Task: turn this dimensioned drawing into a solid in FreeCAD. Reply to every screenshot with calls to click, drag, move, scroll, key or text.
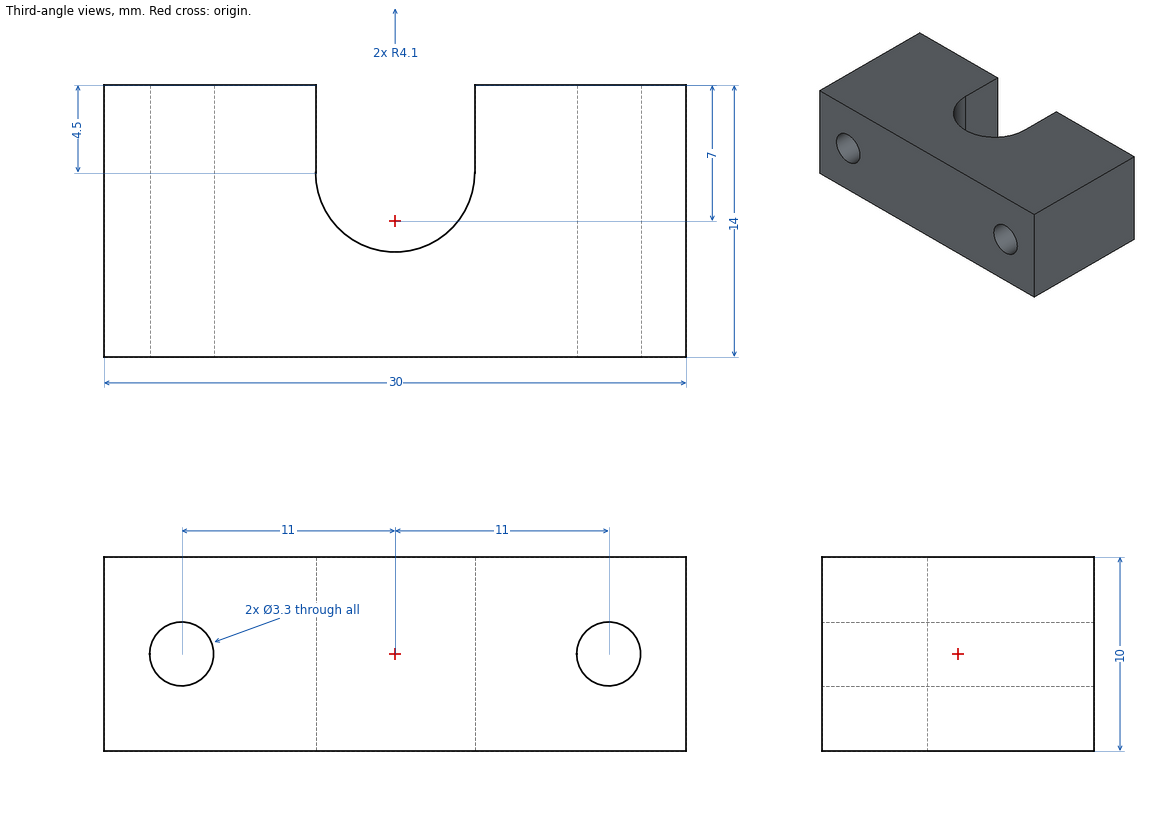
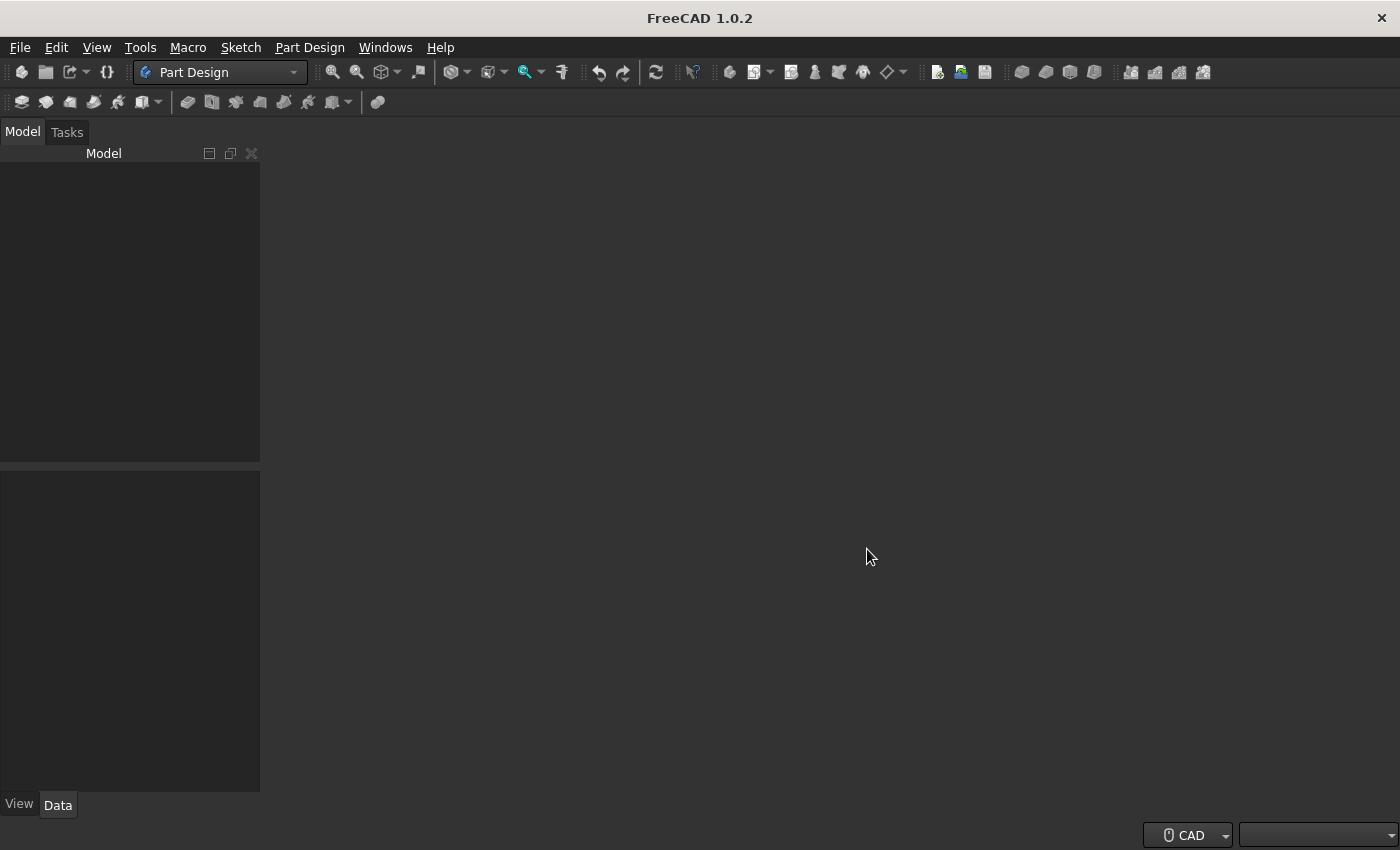
click(938, 72)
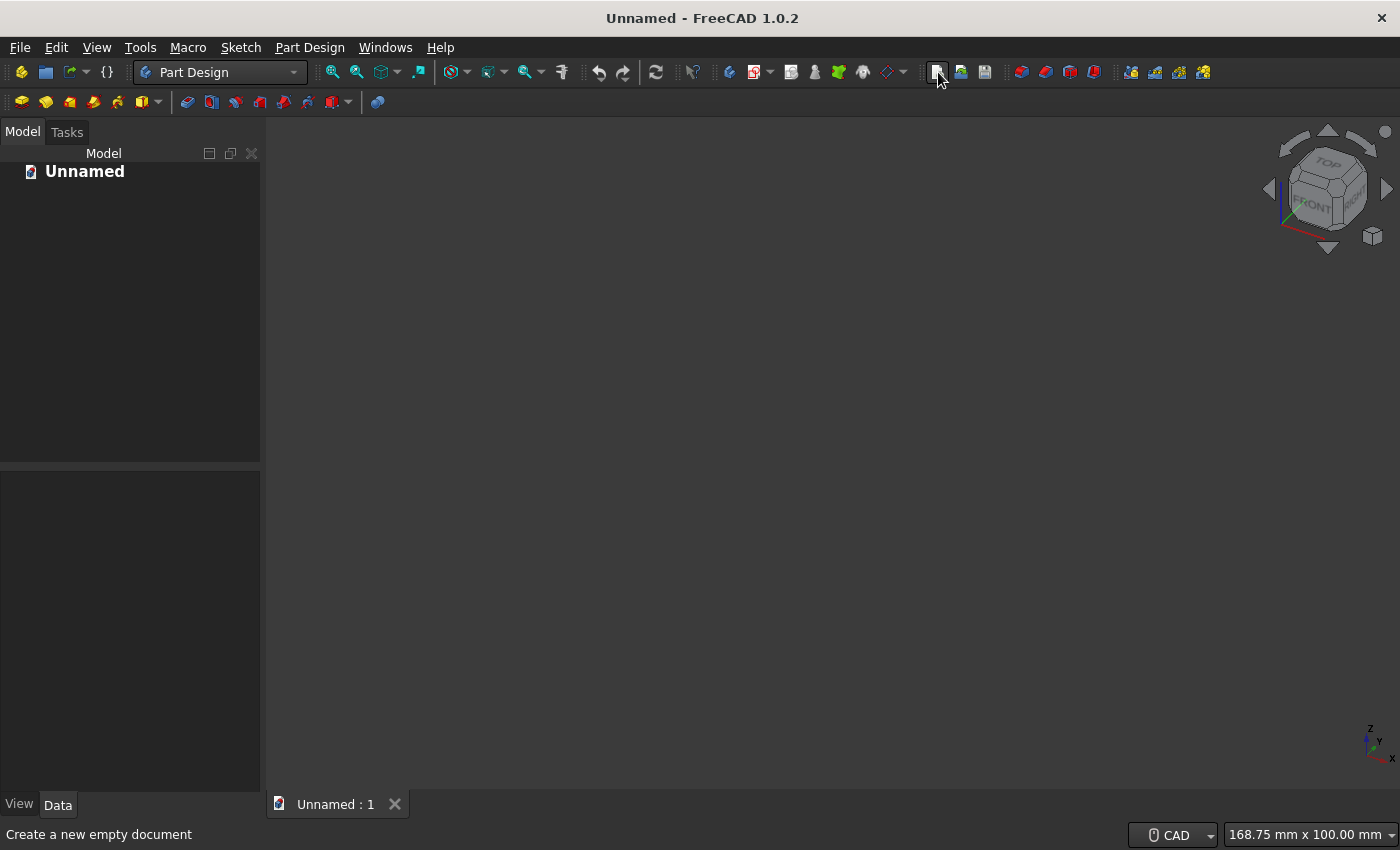
click(754, 72)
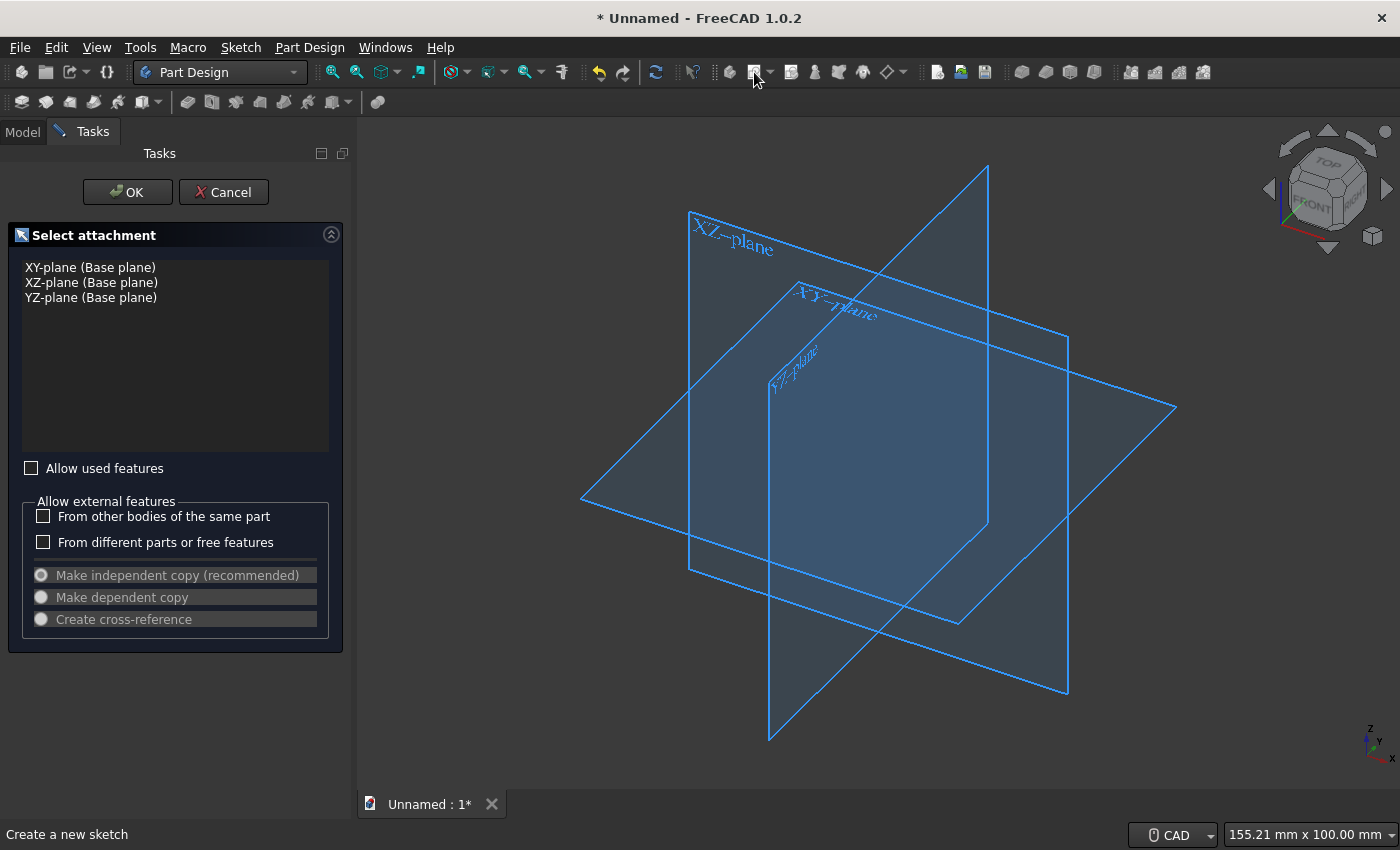
click(82, 268)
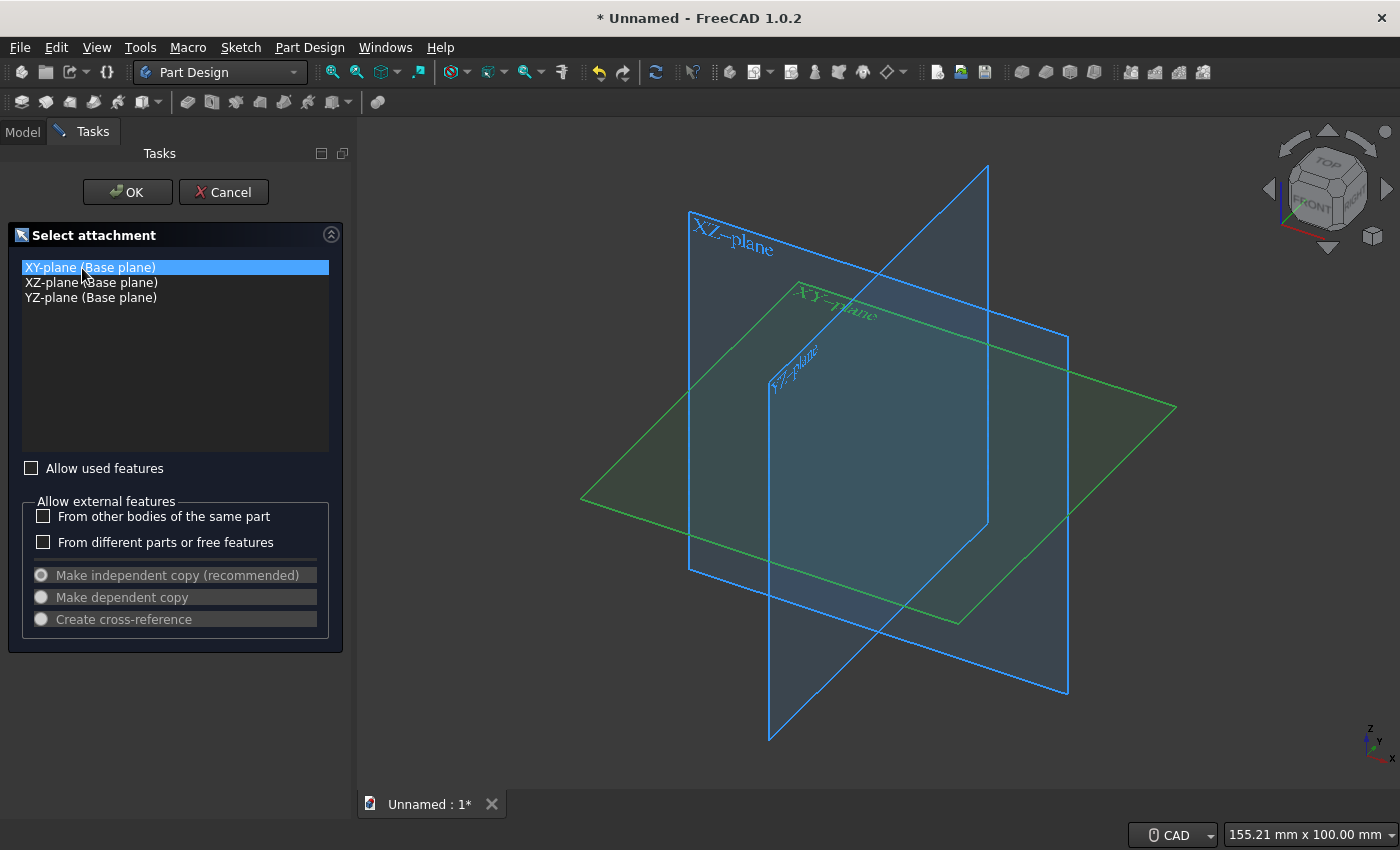
click(128, 192)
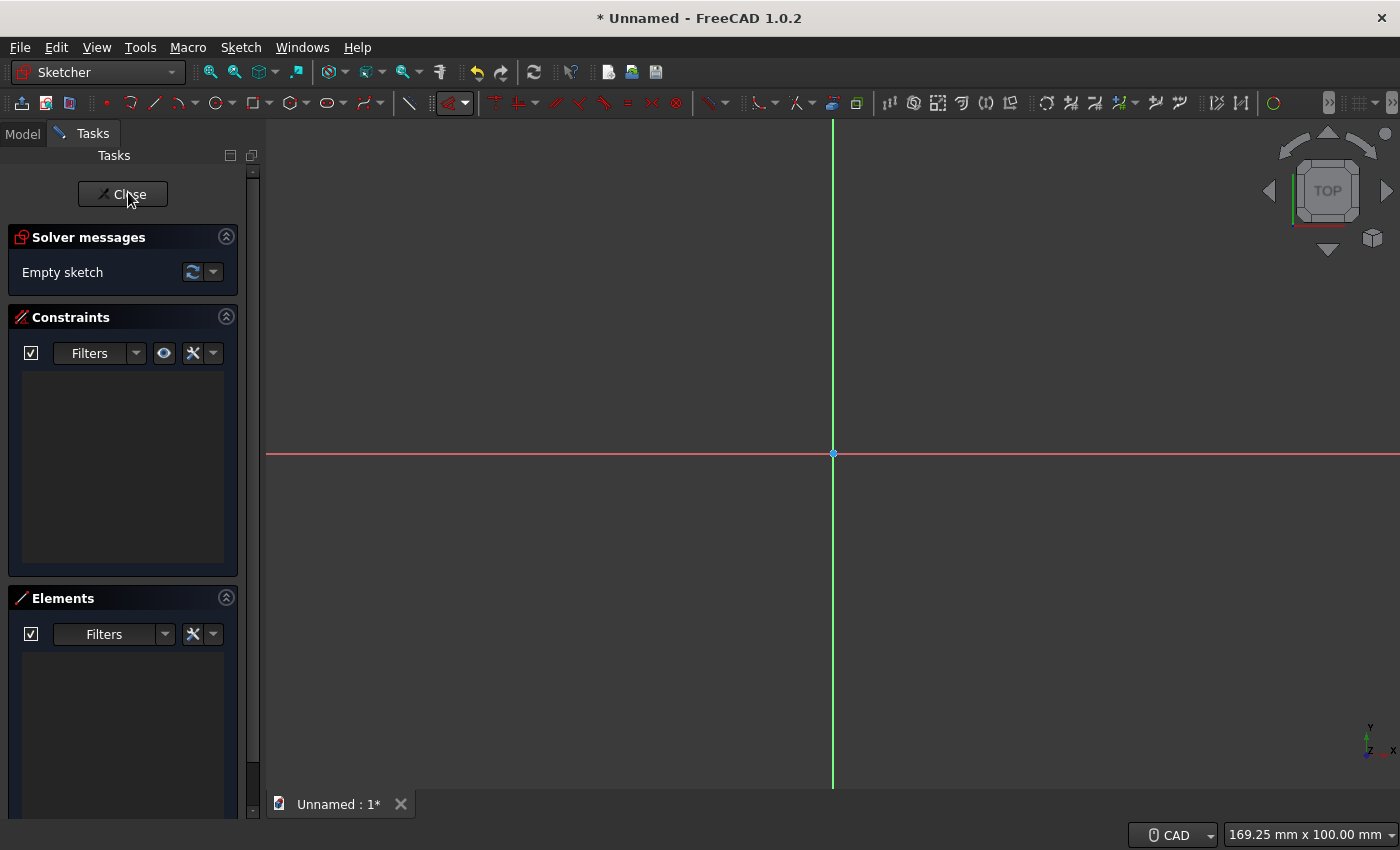
scroll(863, 454, up, 6)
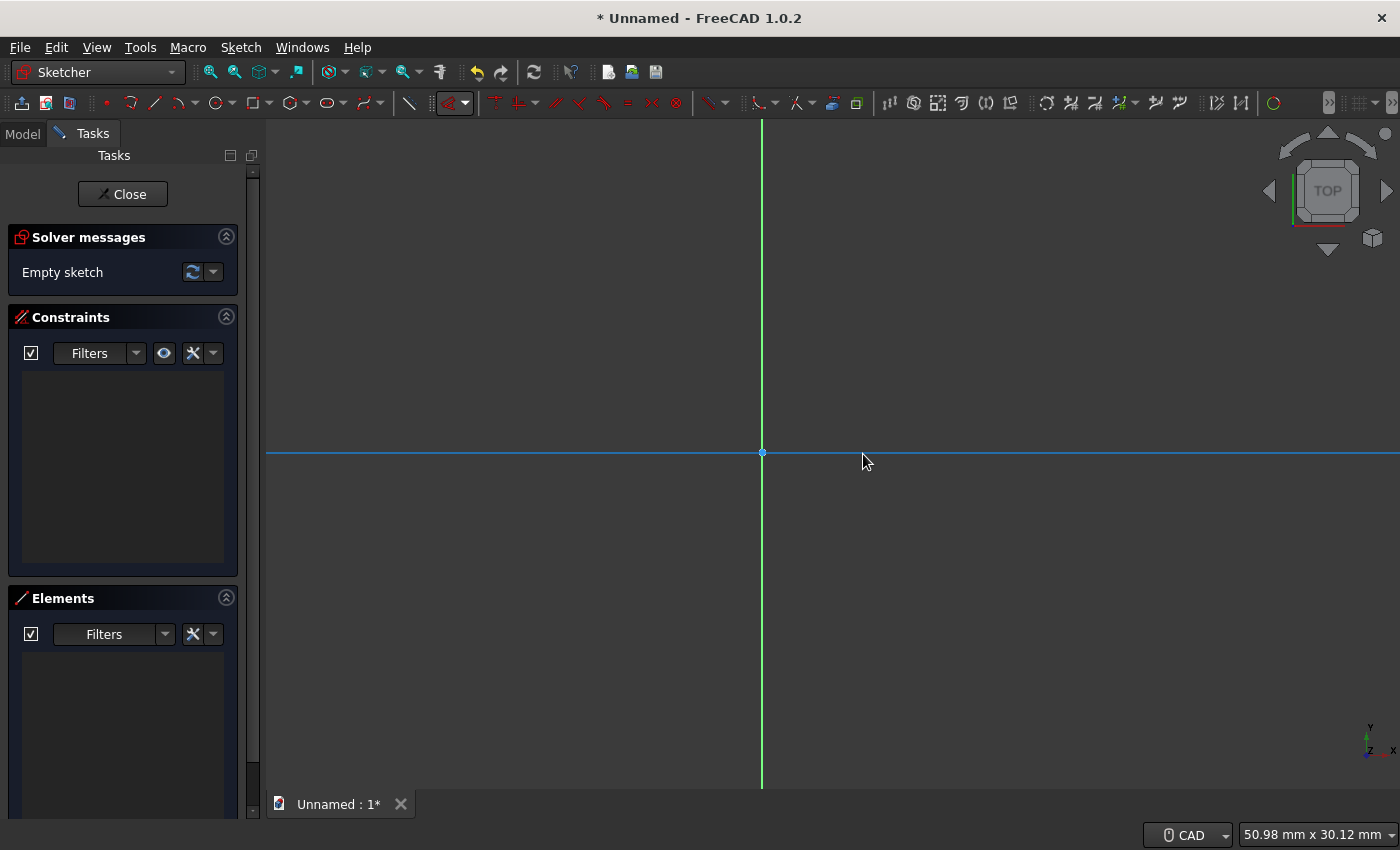
click(272, 104)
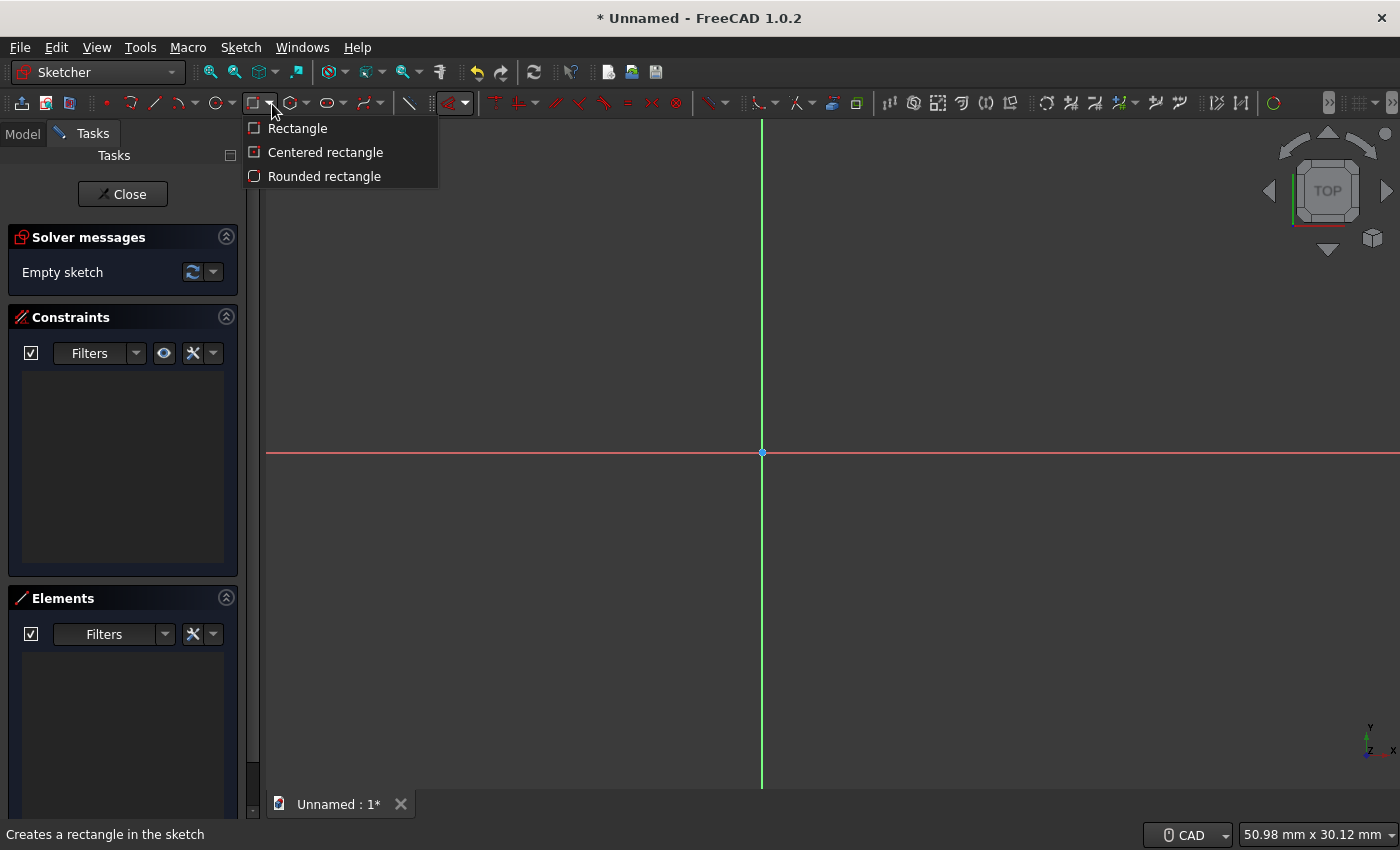
click(340, 152)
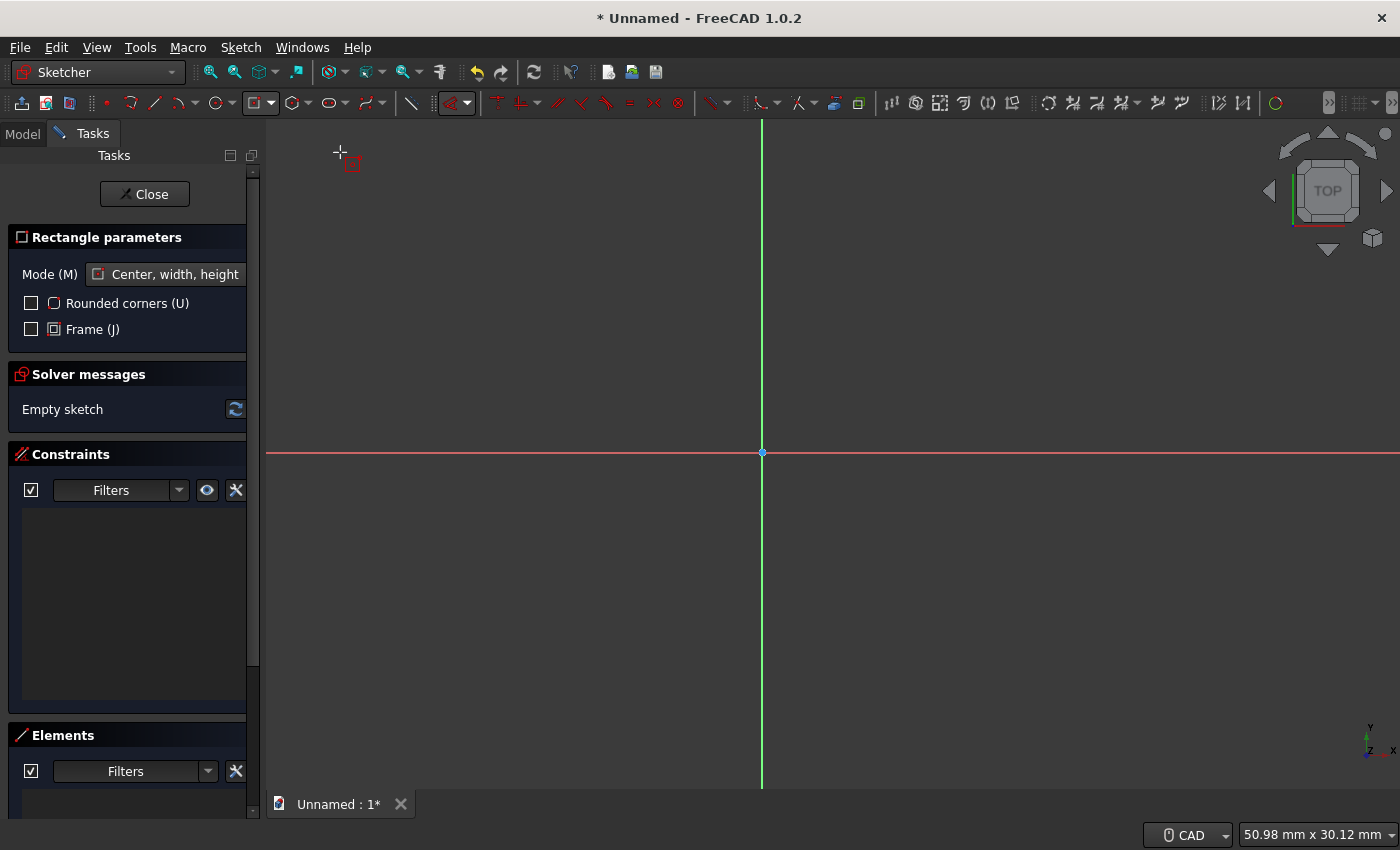
click(762, 453)
move(1096, 297)